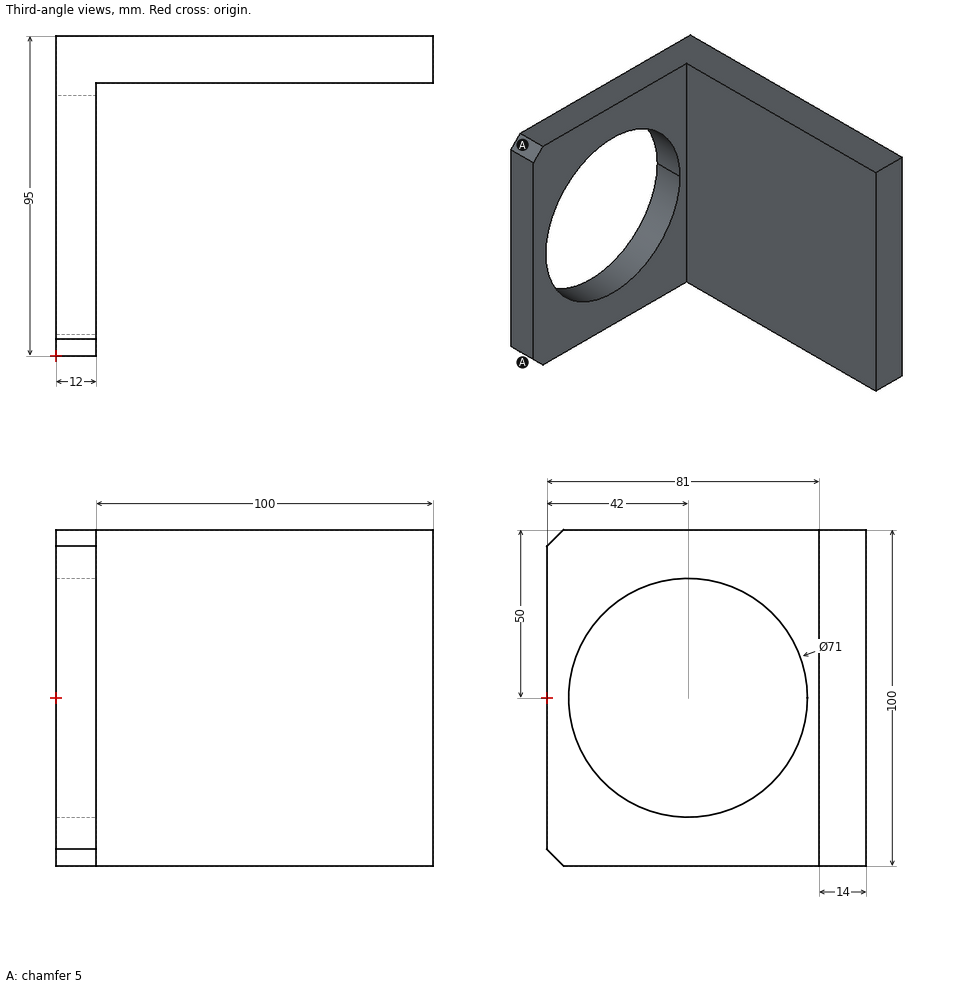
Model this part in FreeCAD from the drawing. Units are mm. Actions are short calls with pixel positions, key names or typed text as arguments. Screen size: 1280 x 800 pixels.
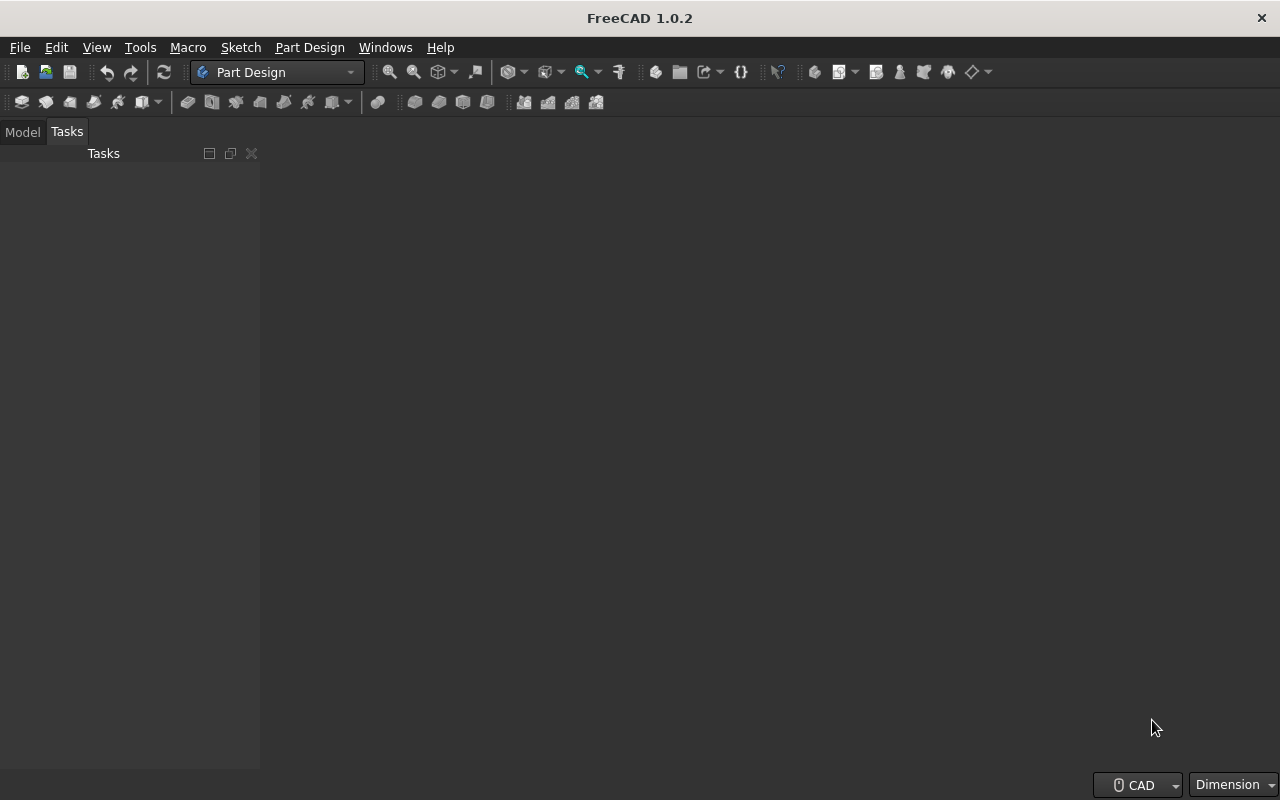
click(22, 72)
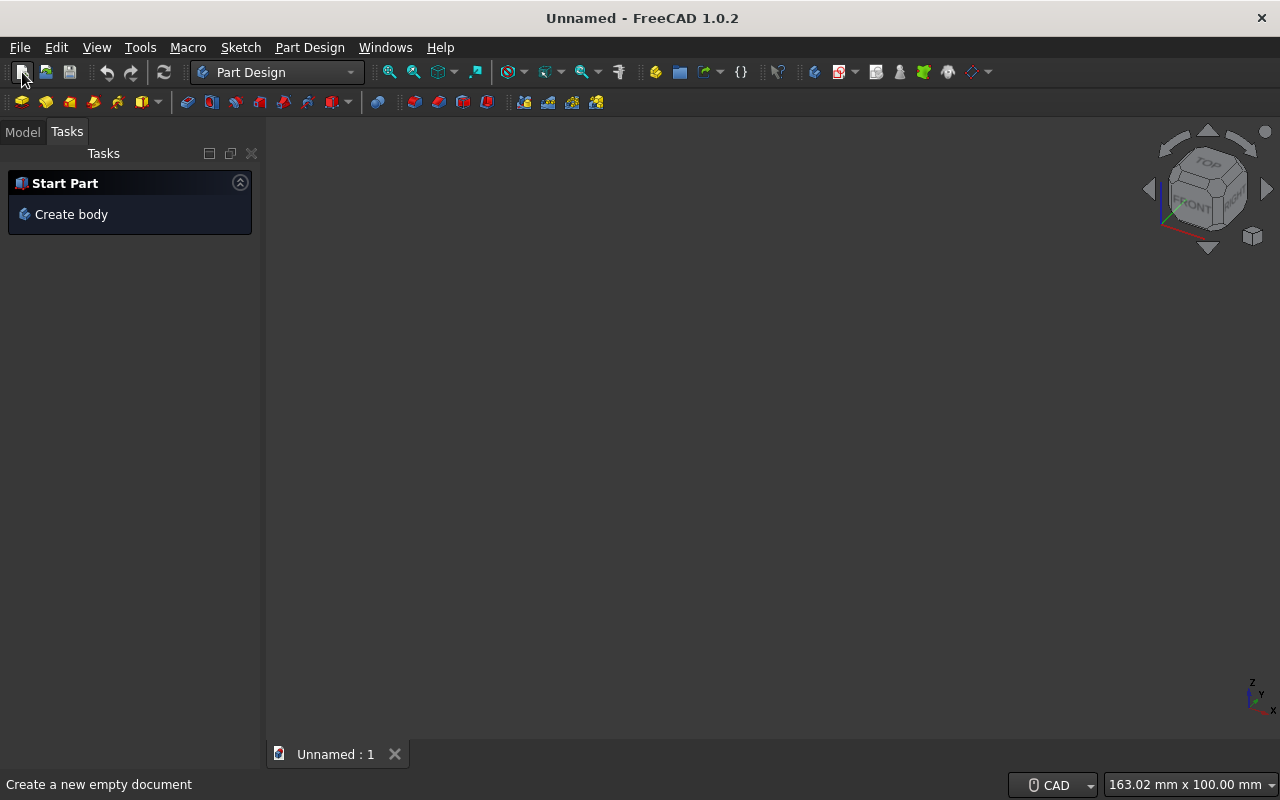
click(840, 72)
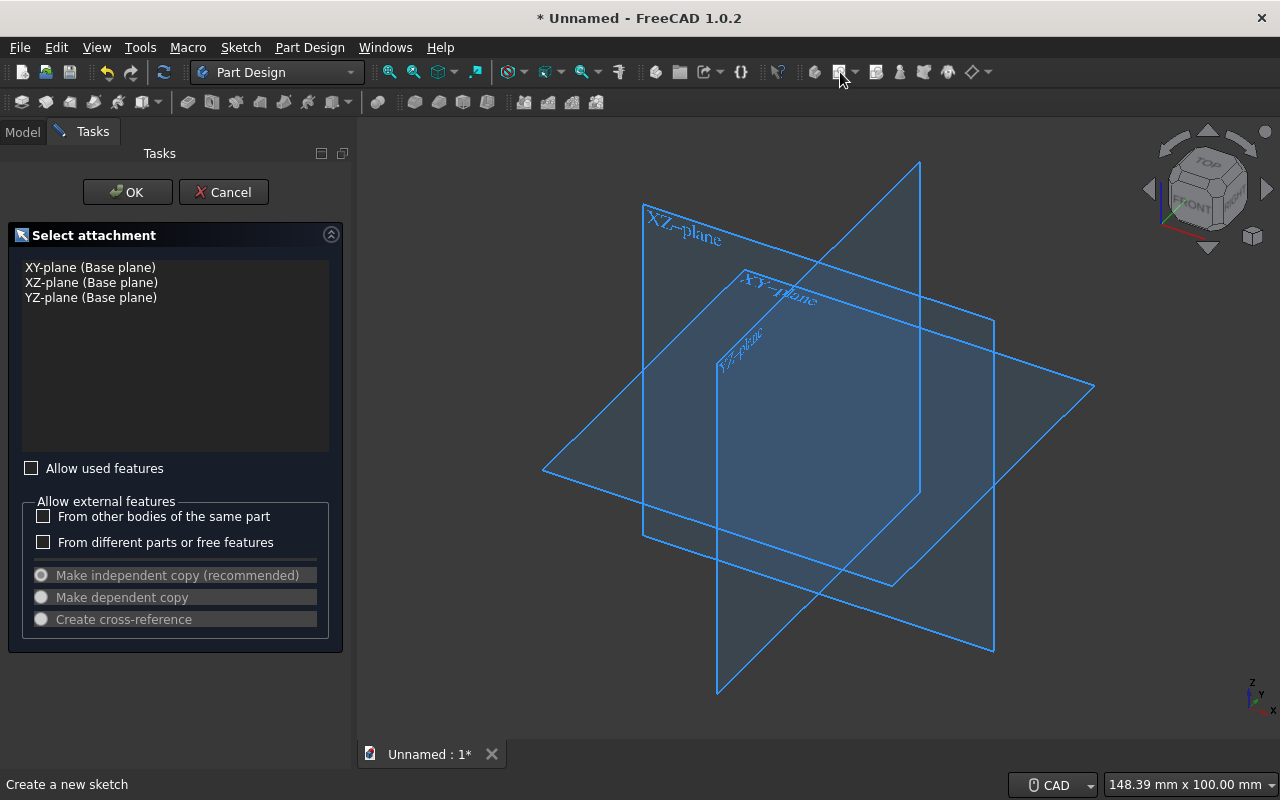
click(82, 268)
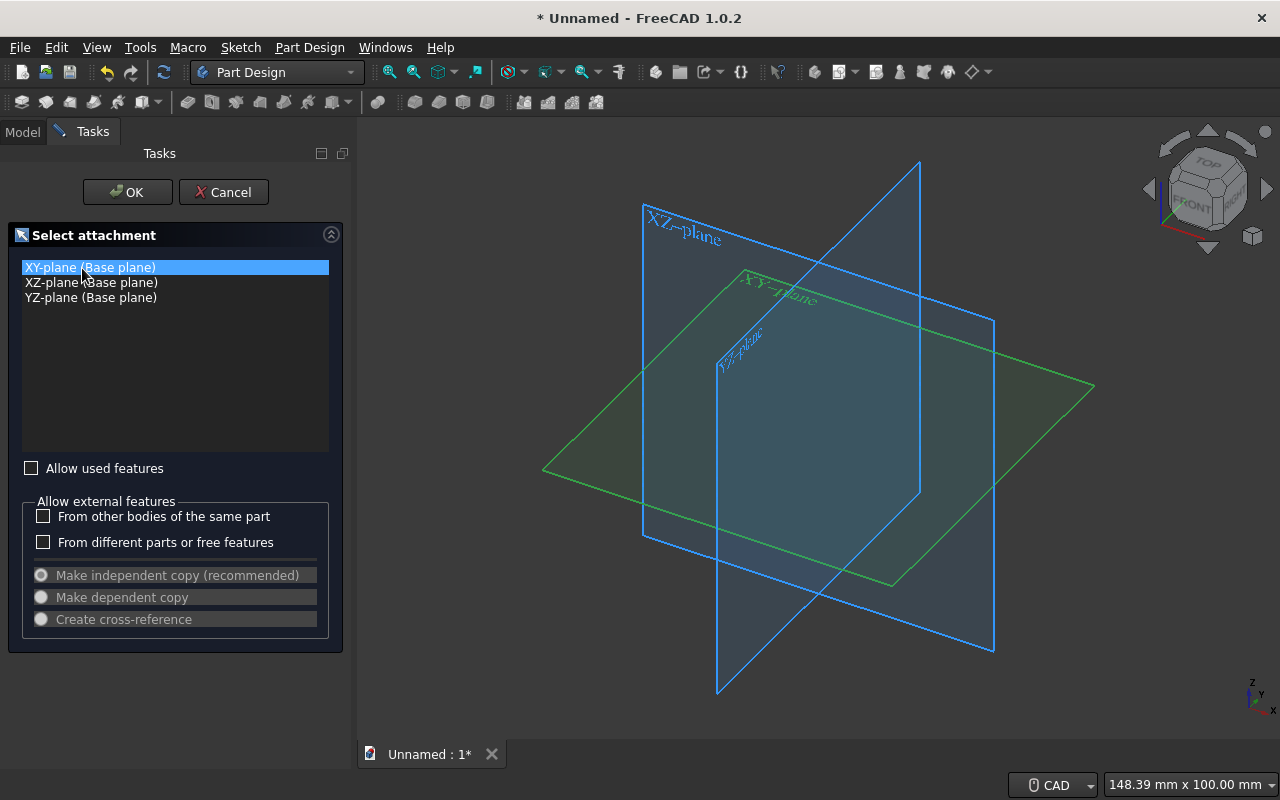
click(128, 192)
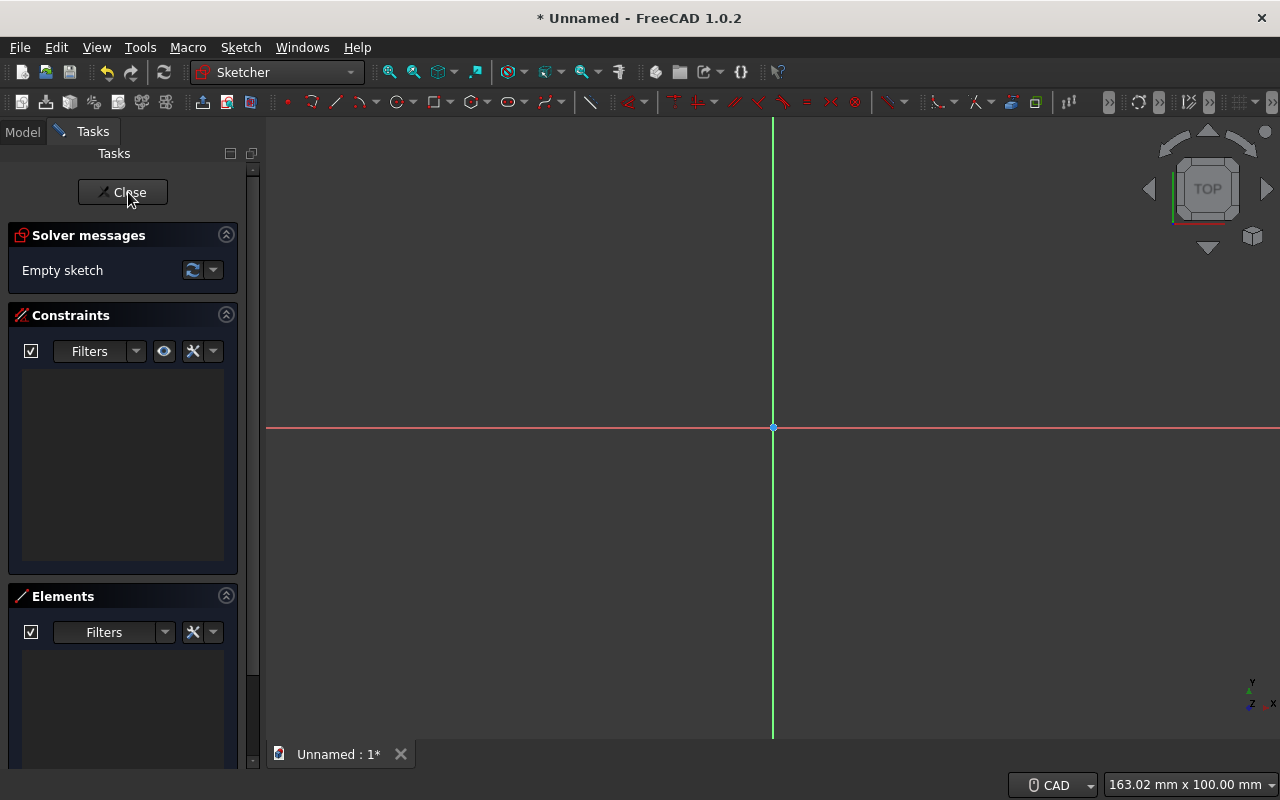
scroll(576, 711, down, 3)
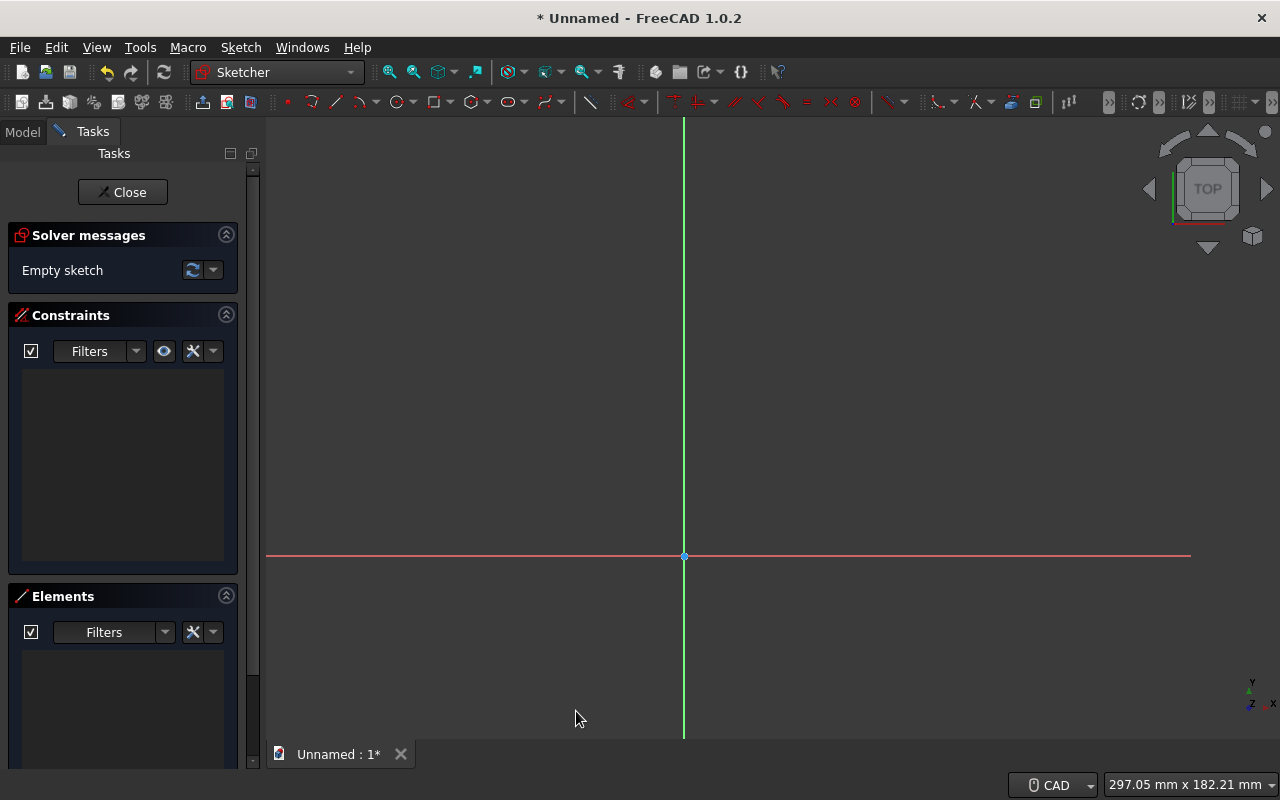
click(434, 102)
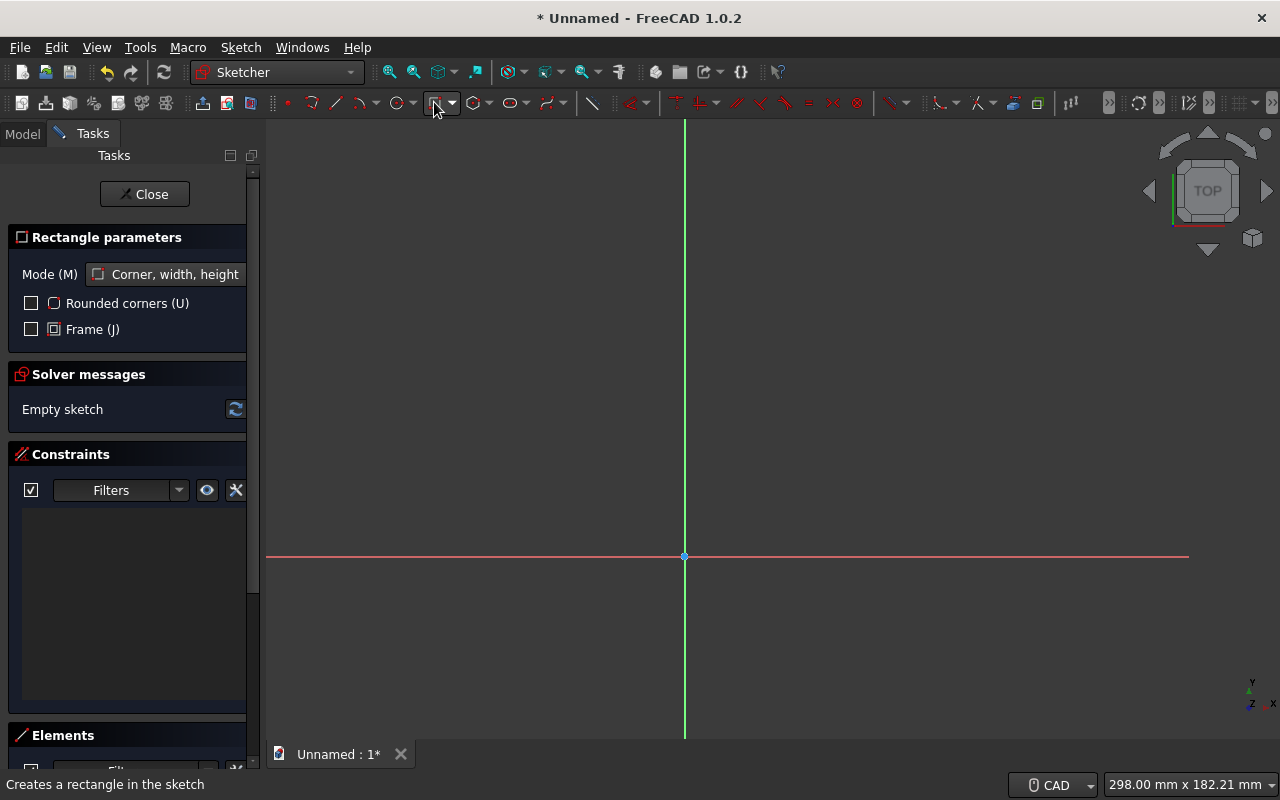
click(685, 557)
move(725, 233)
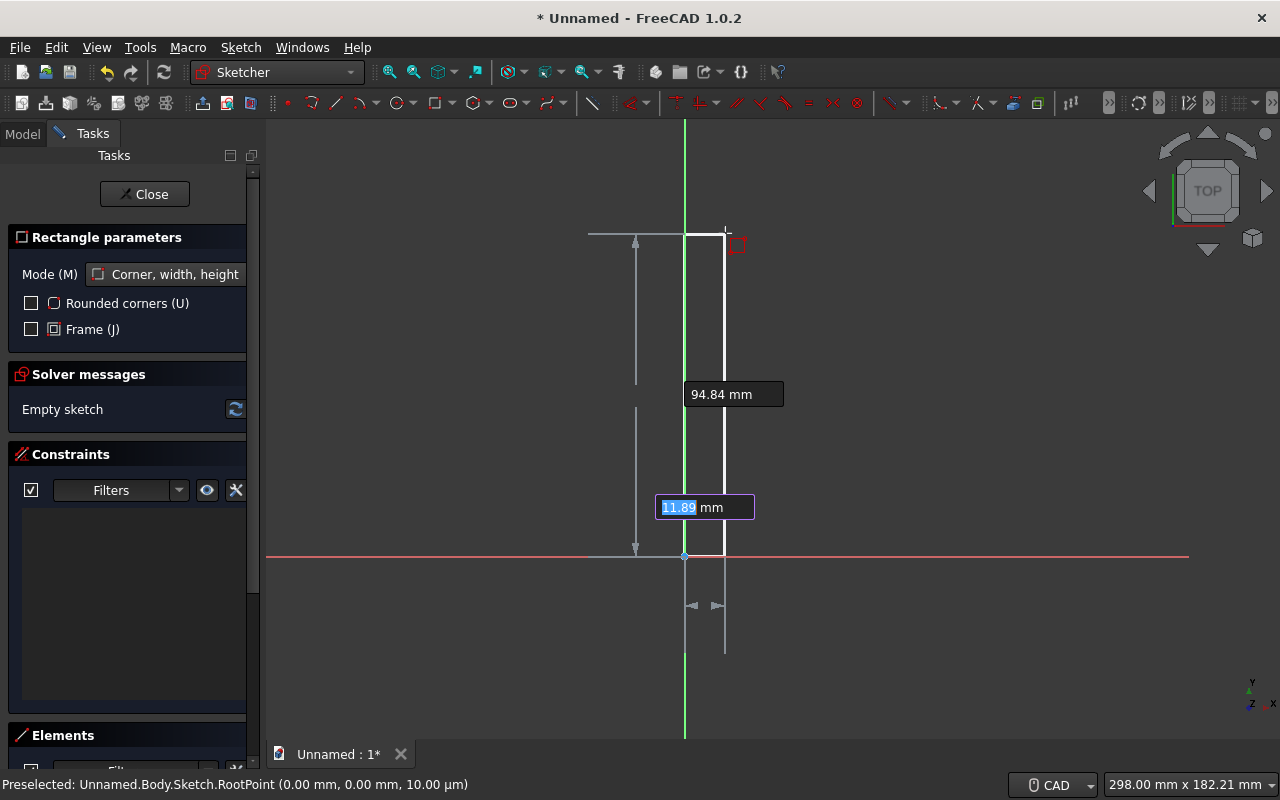
text(12)
key(Tab)
text(95)
key(Return)
key(Escape)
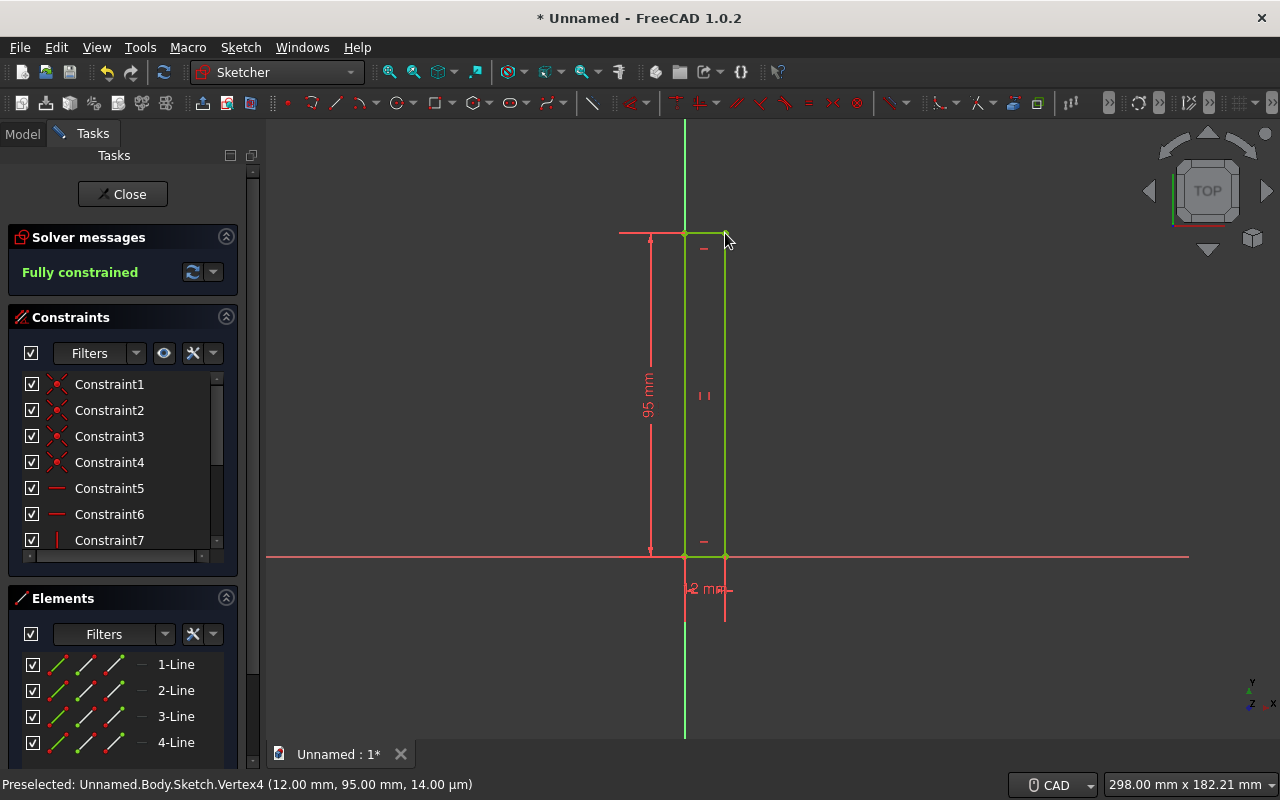
click(123, 194)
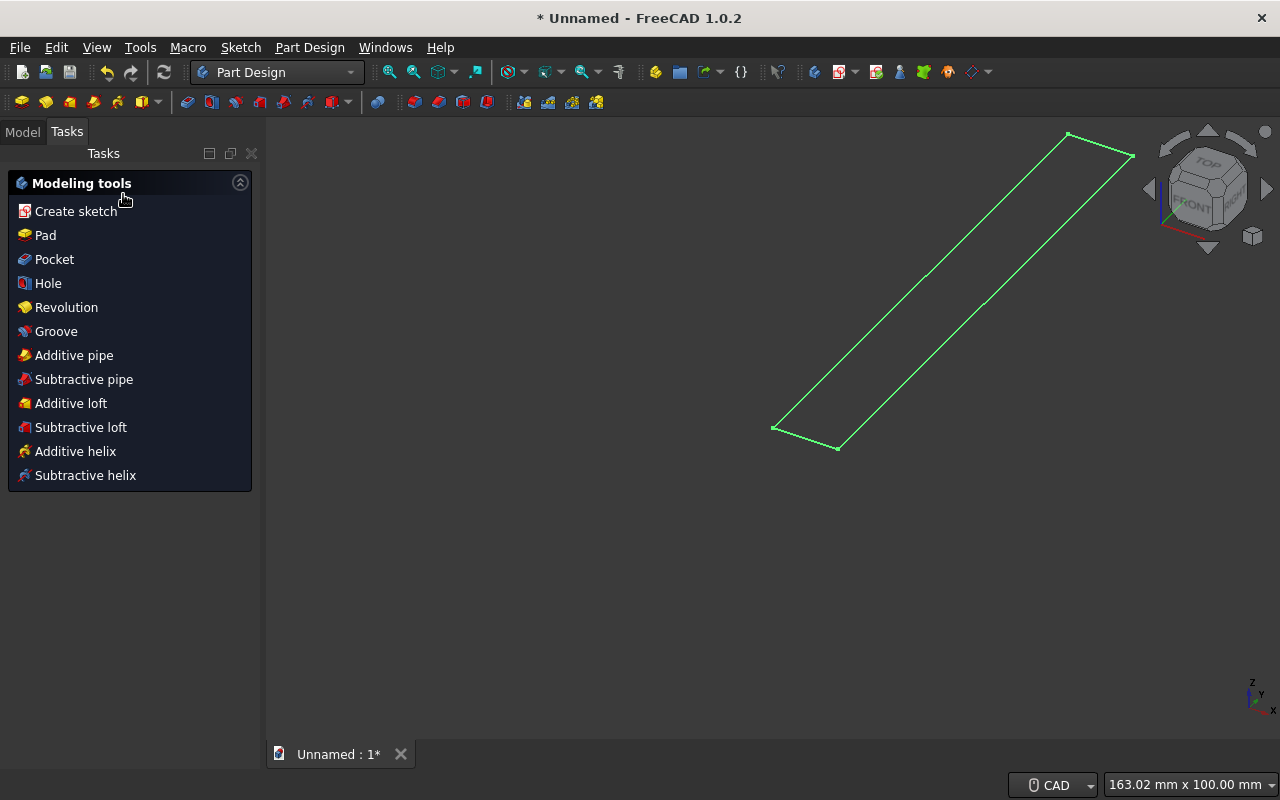
click(22, 102)